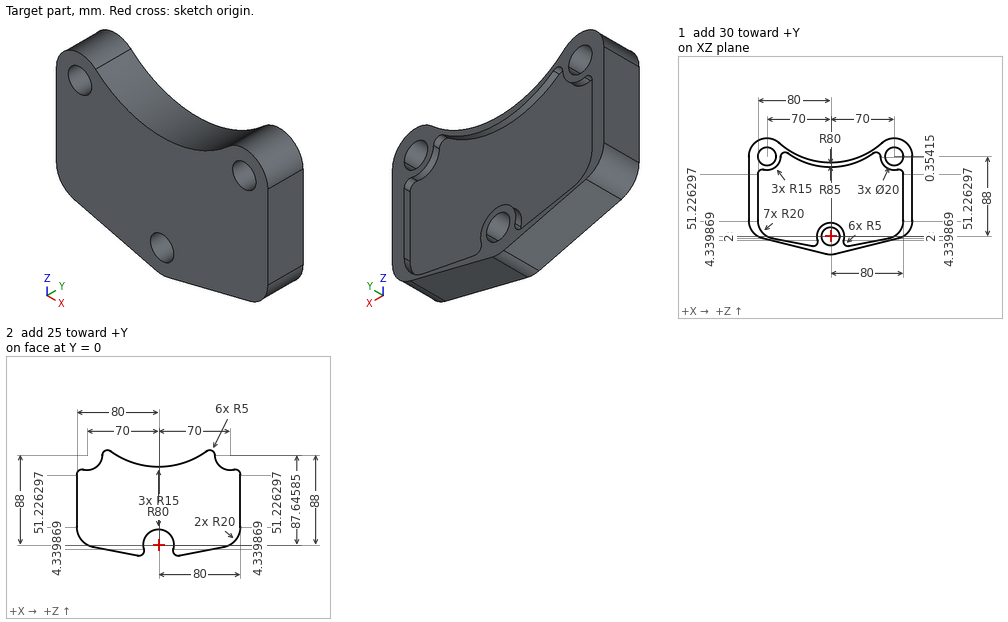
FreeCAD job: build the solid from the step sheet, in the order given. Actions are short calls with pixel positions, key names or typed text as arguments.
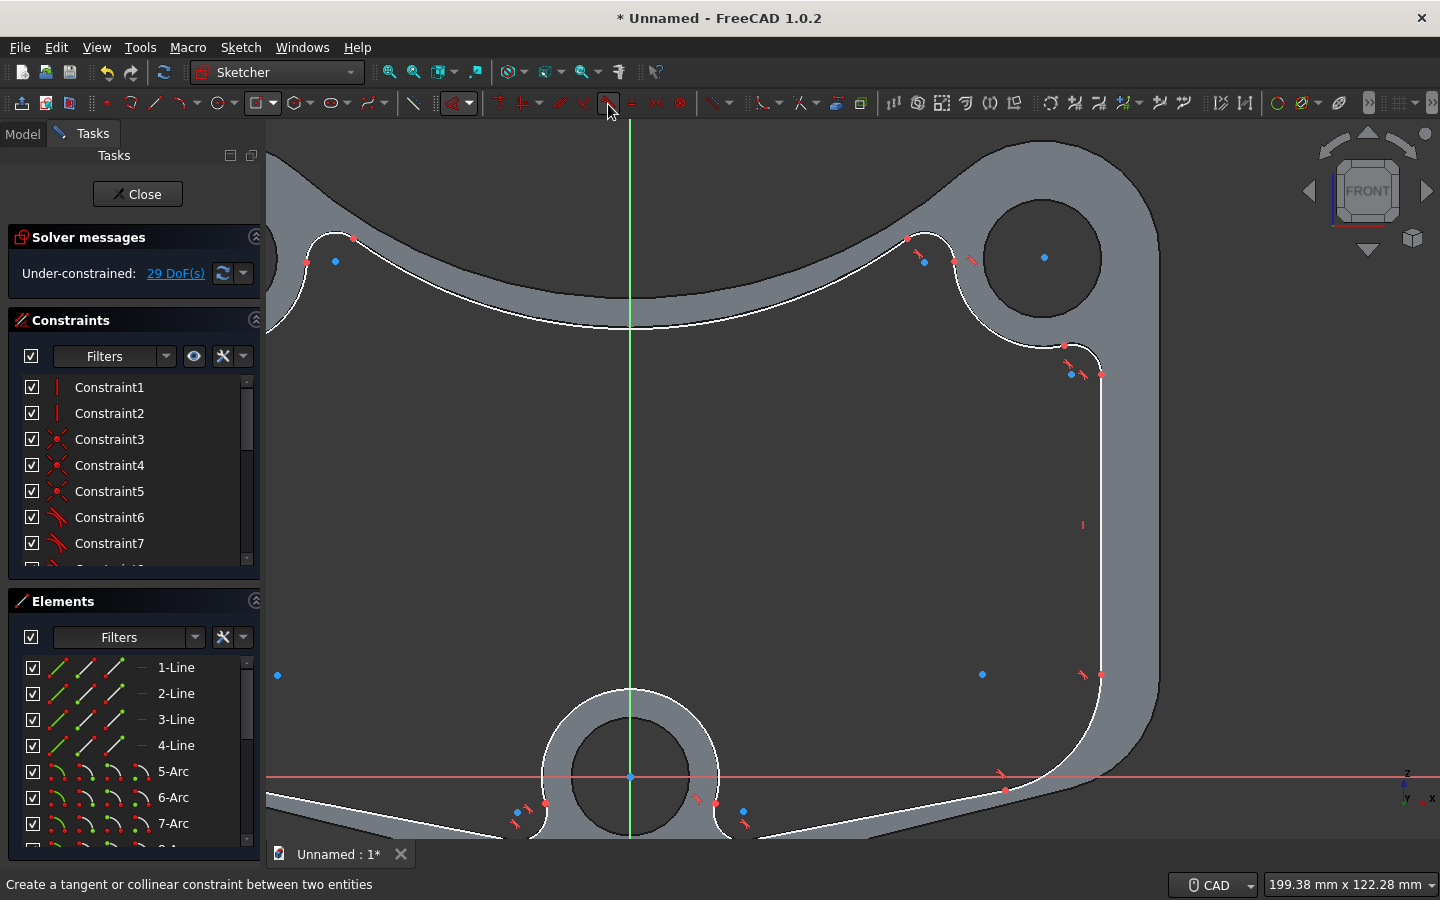
click(513, 314)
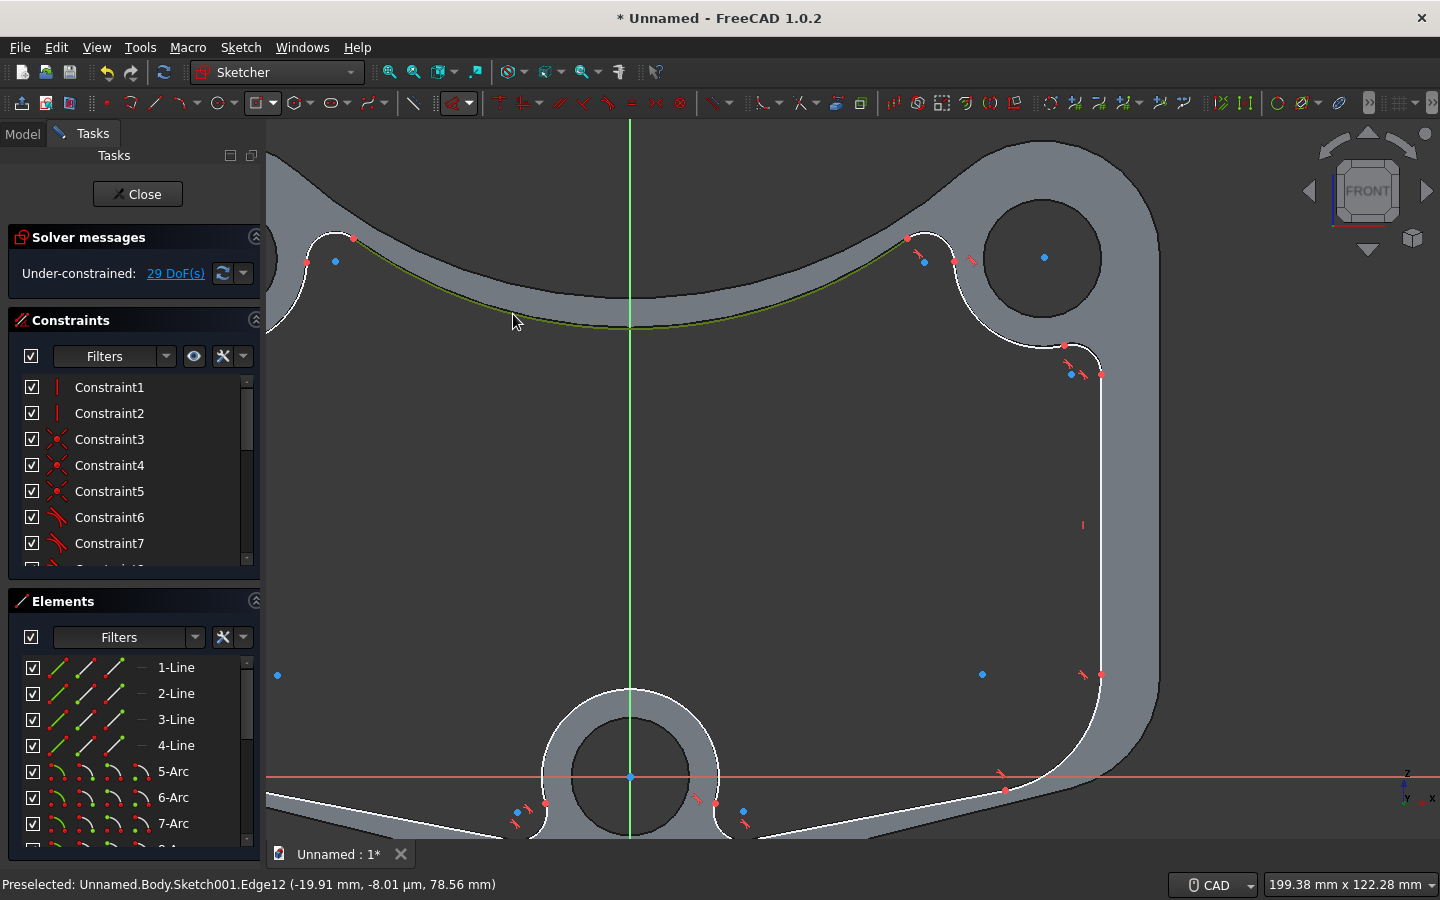
click(335, 233)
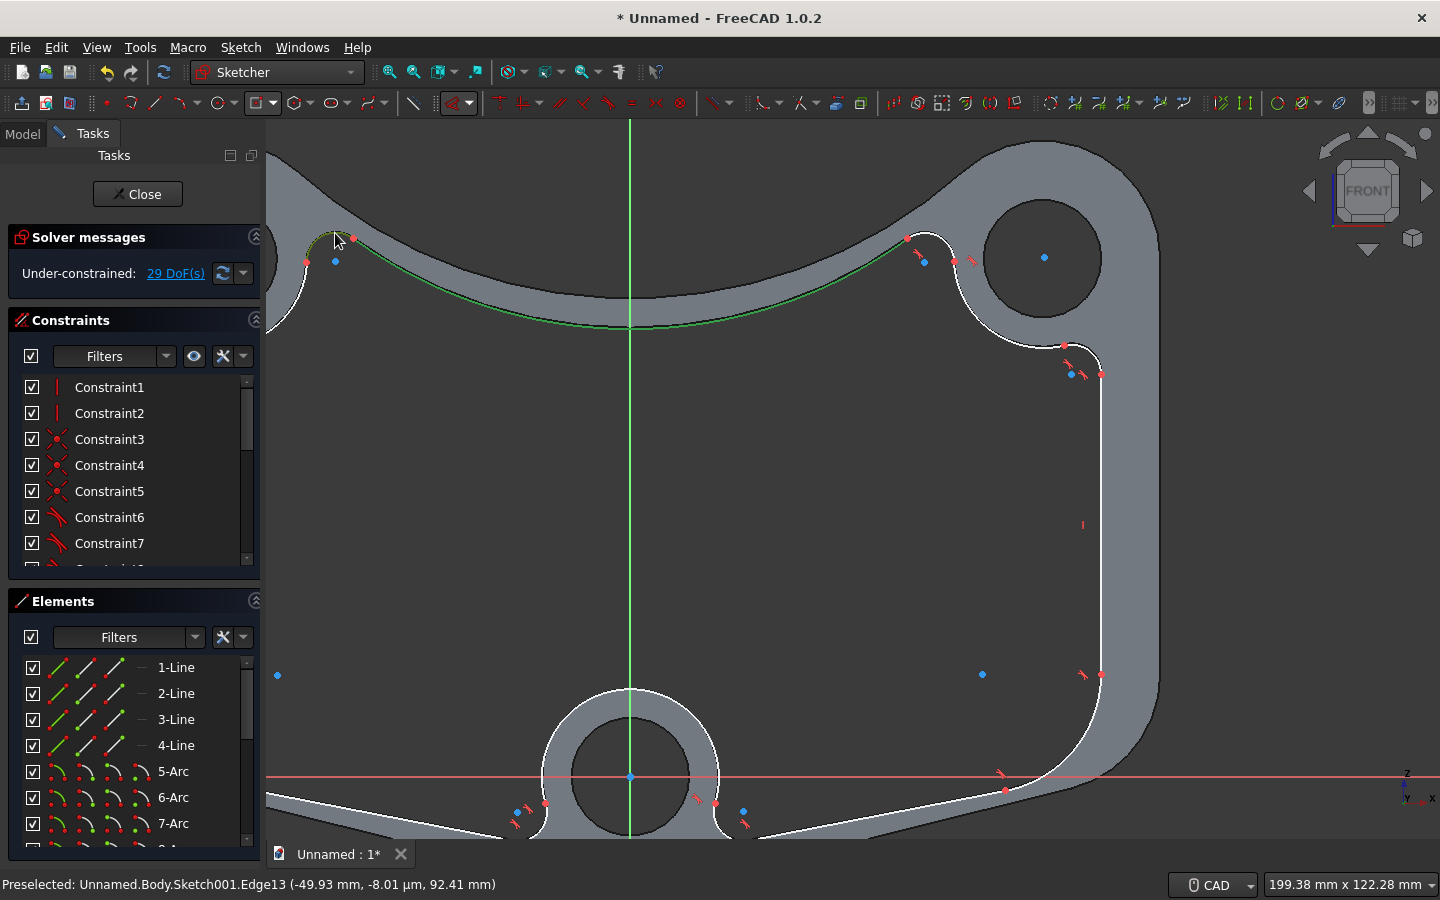
click(608, 104)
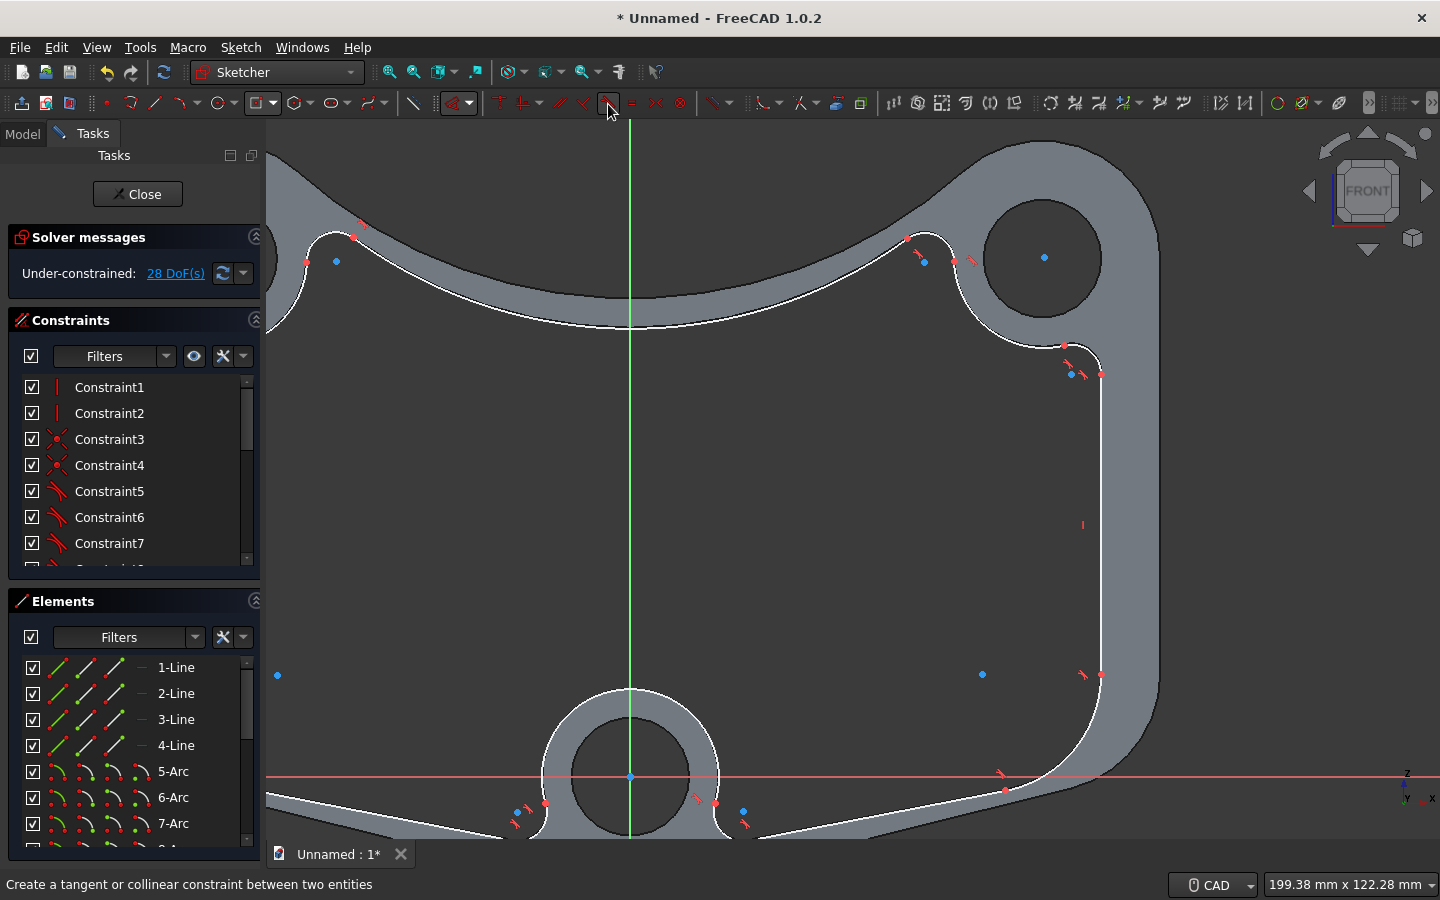
click(335, 232)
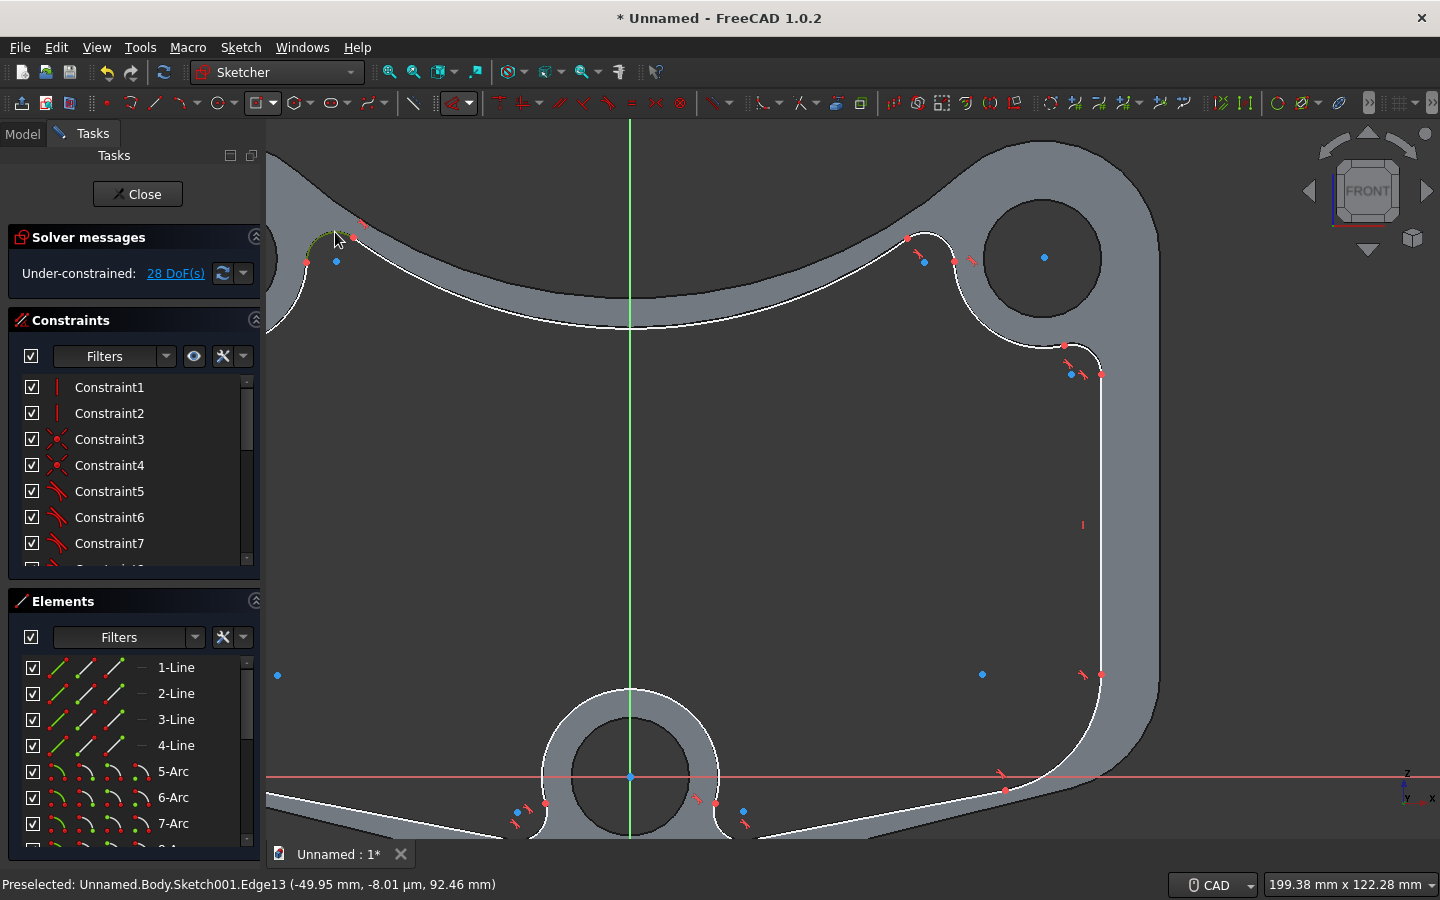
click(300, 293)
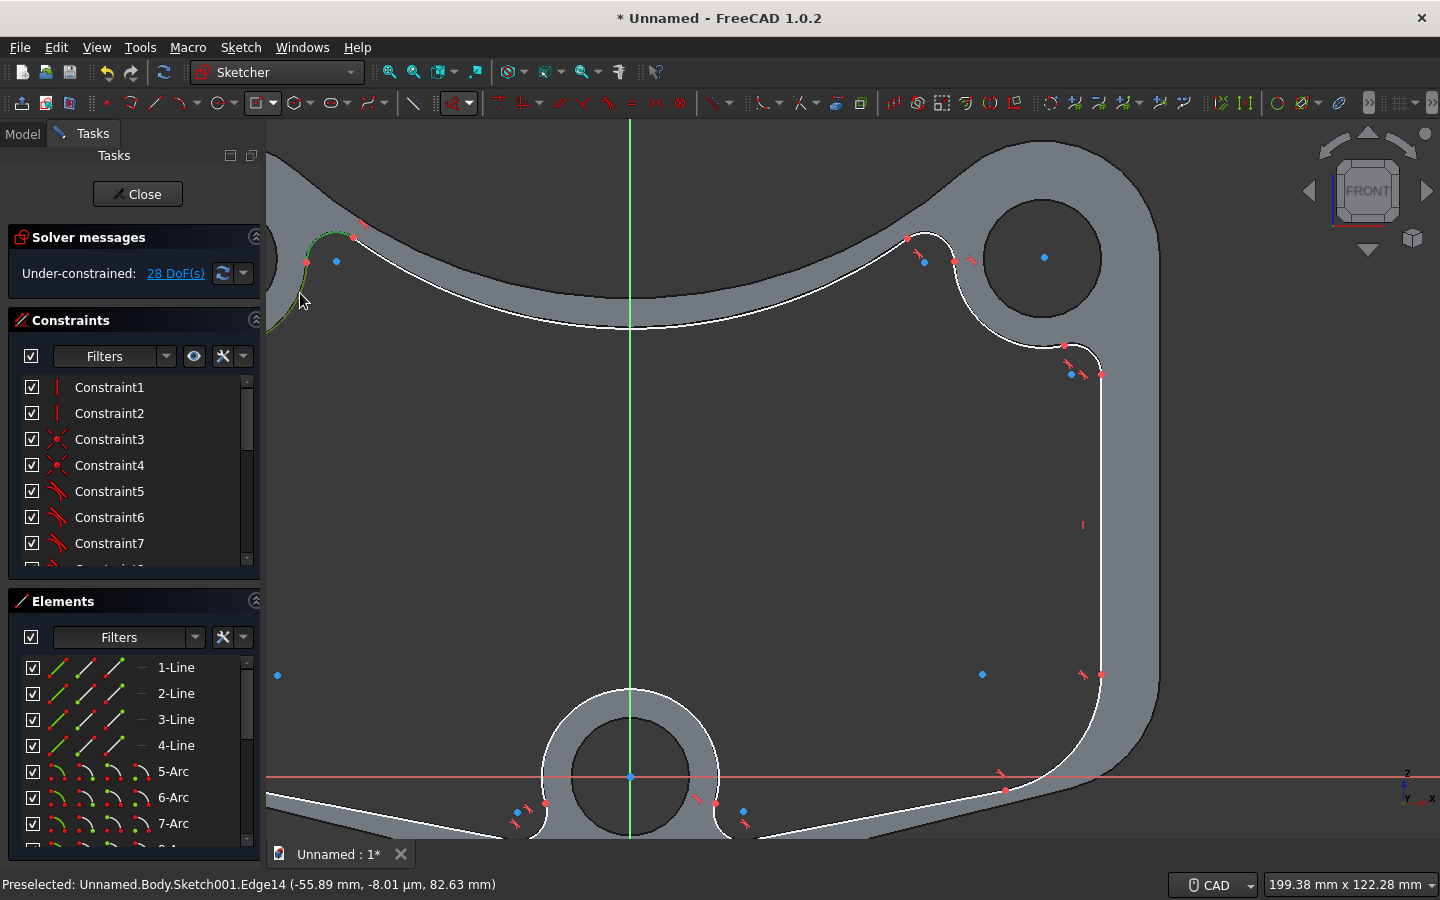
click(608, 104)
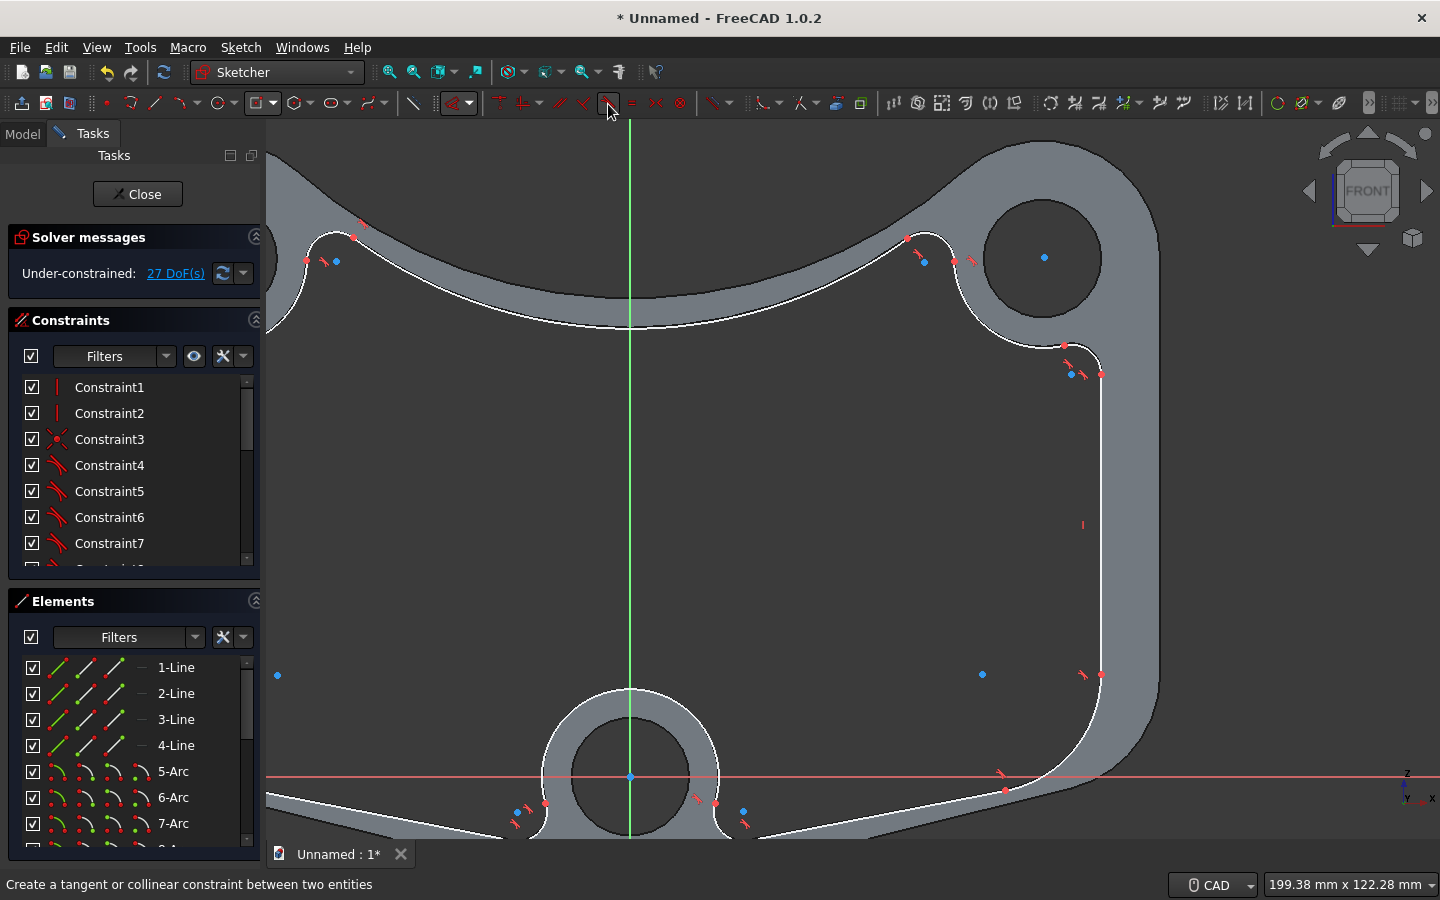
click(301, 292)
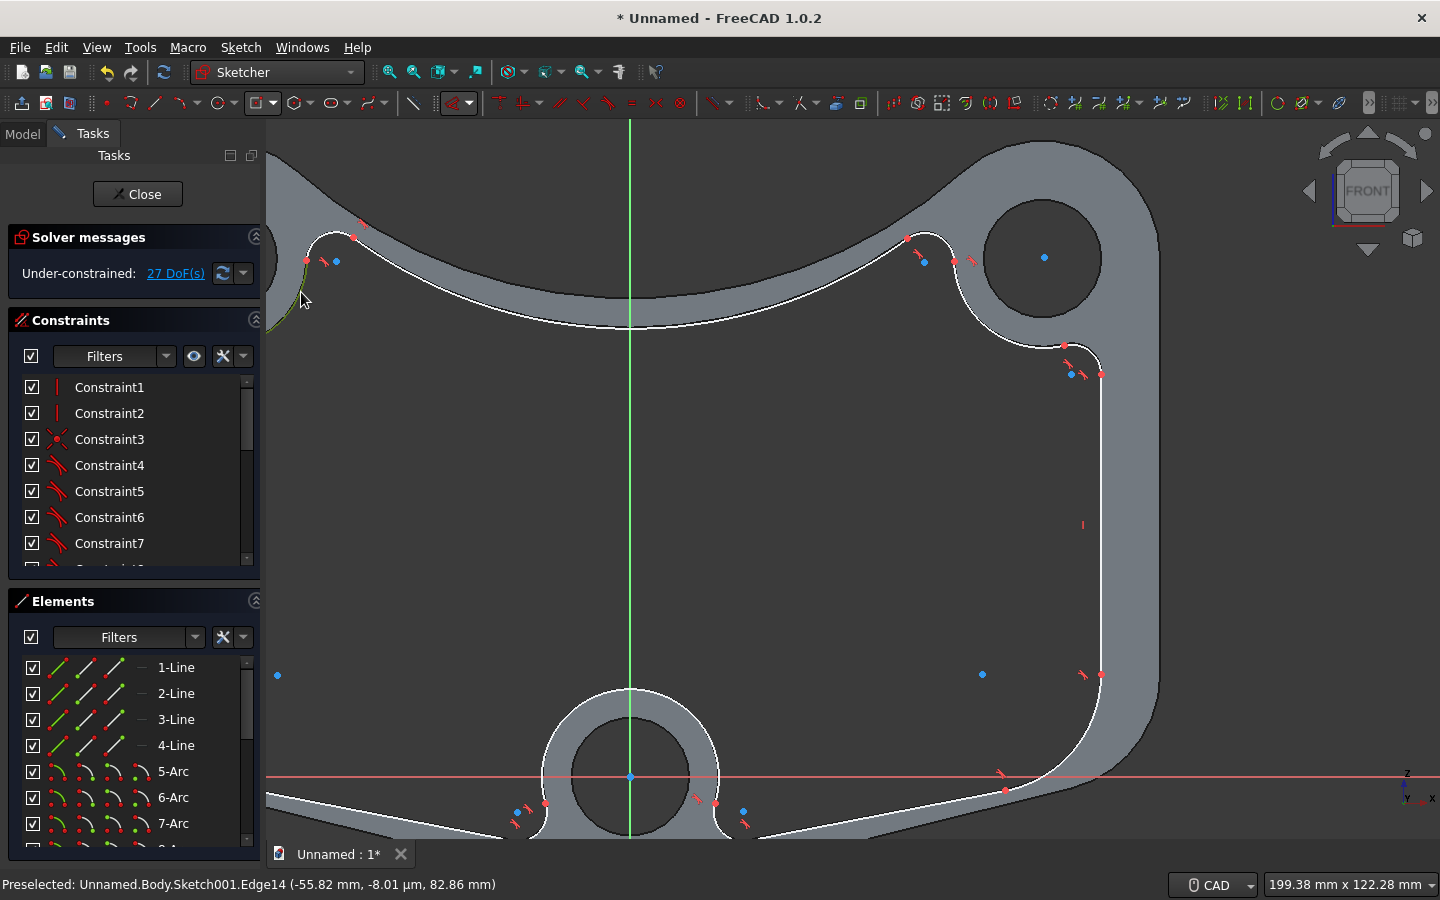
scroll(1098, 360, down, 2)